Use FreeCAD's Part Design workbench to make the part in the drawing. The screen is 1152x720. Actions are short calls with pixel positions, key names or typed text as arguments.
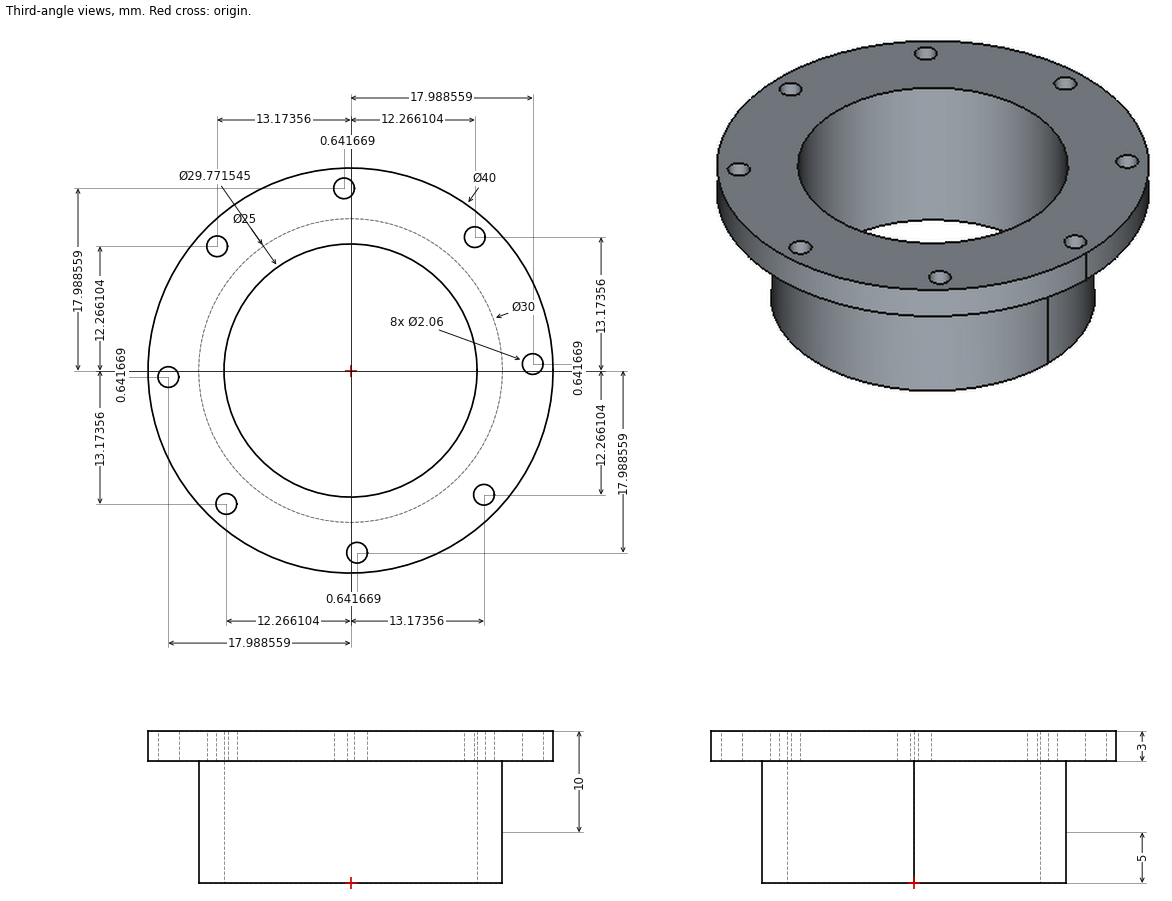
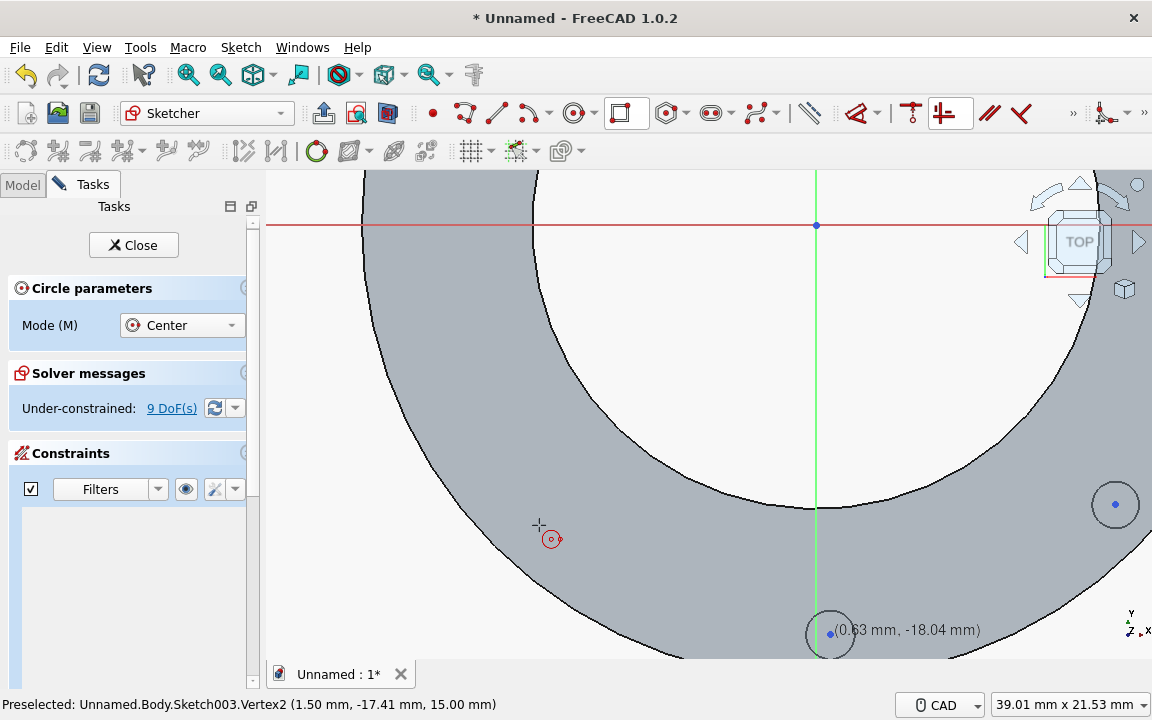
click(538, 524)
click(554, 508)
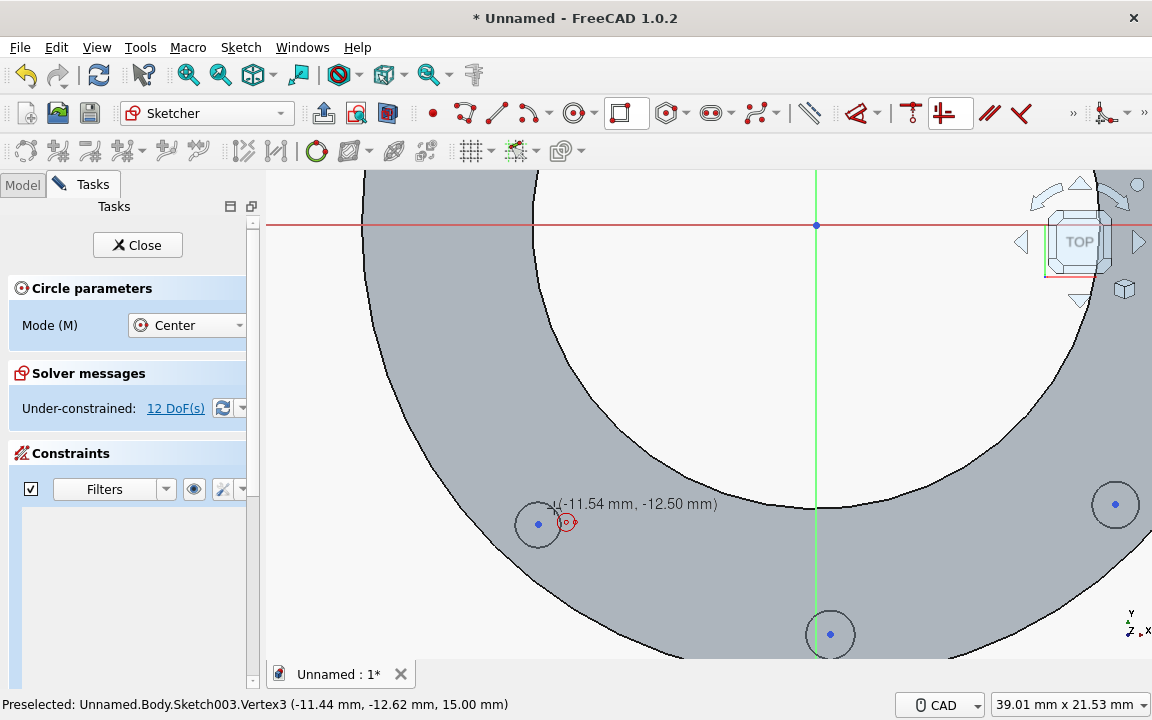
click(408, 240)
click(424, 256)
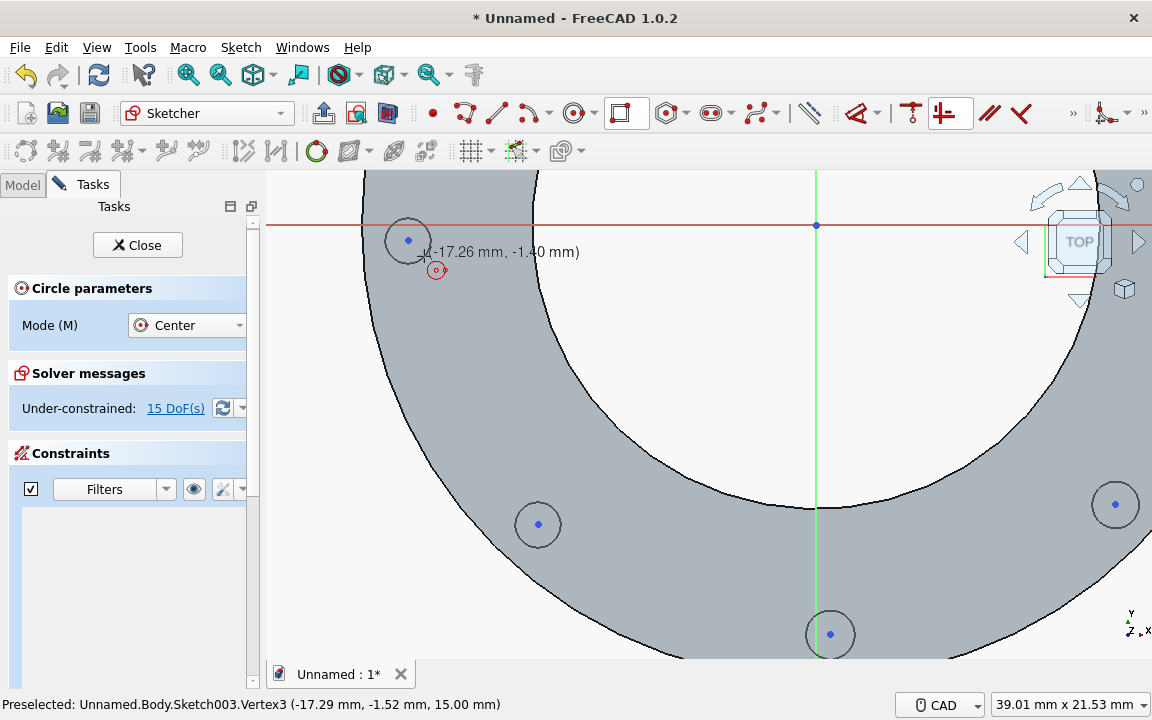
scroll(538, 525, down, 5)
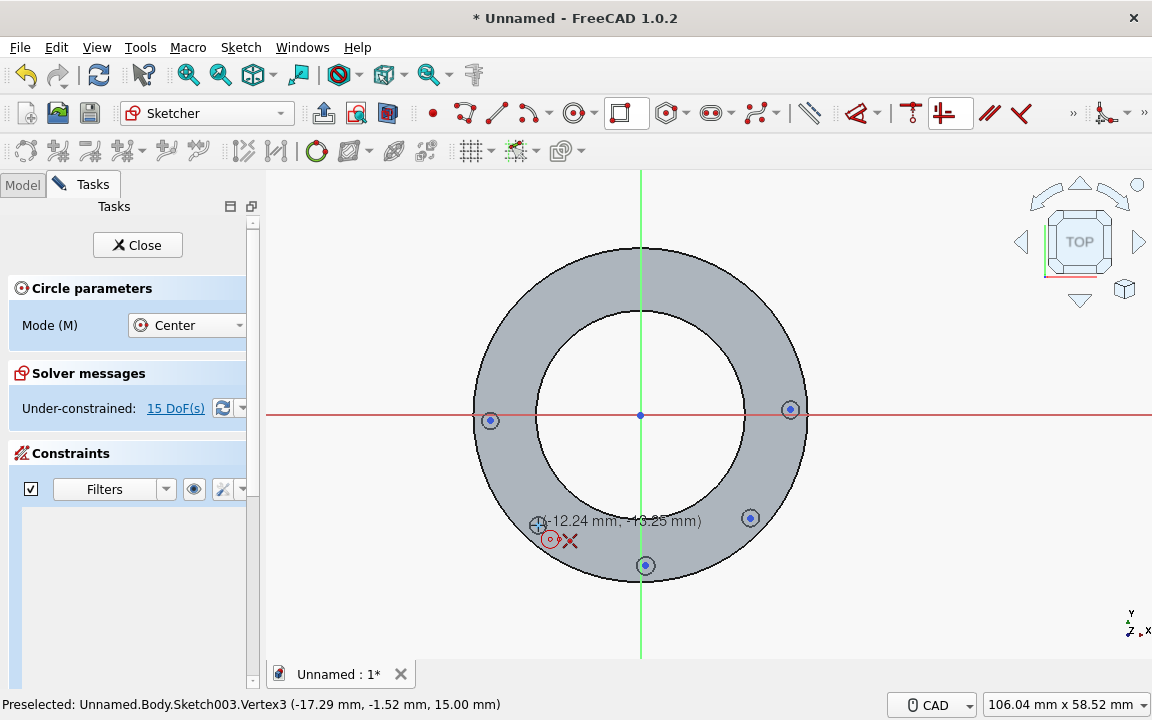
scroll(530, 313, up, 5)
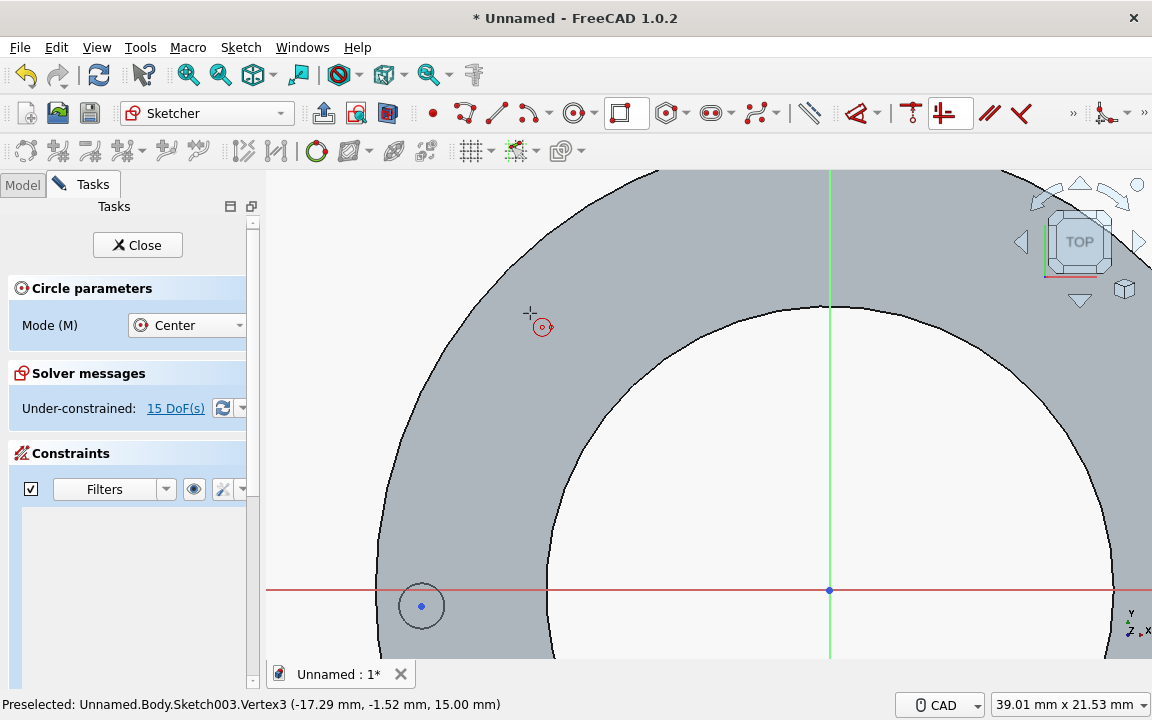
click(531, 312)
click(547, 295)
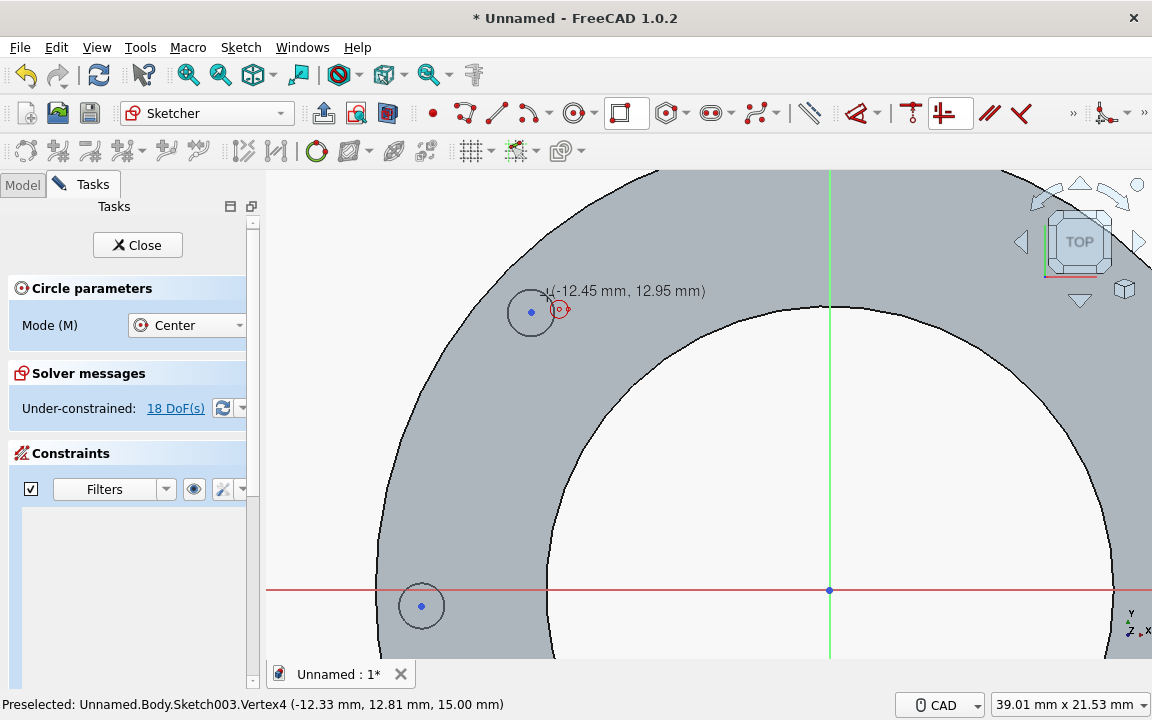
scroll(530, 312, down, 5)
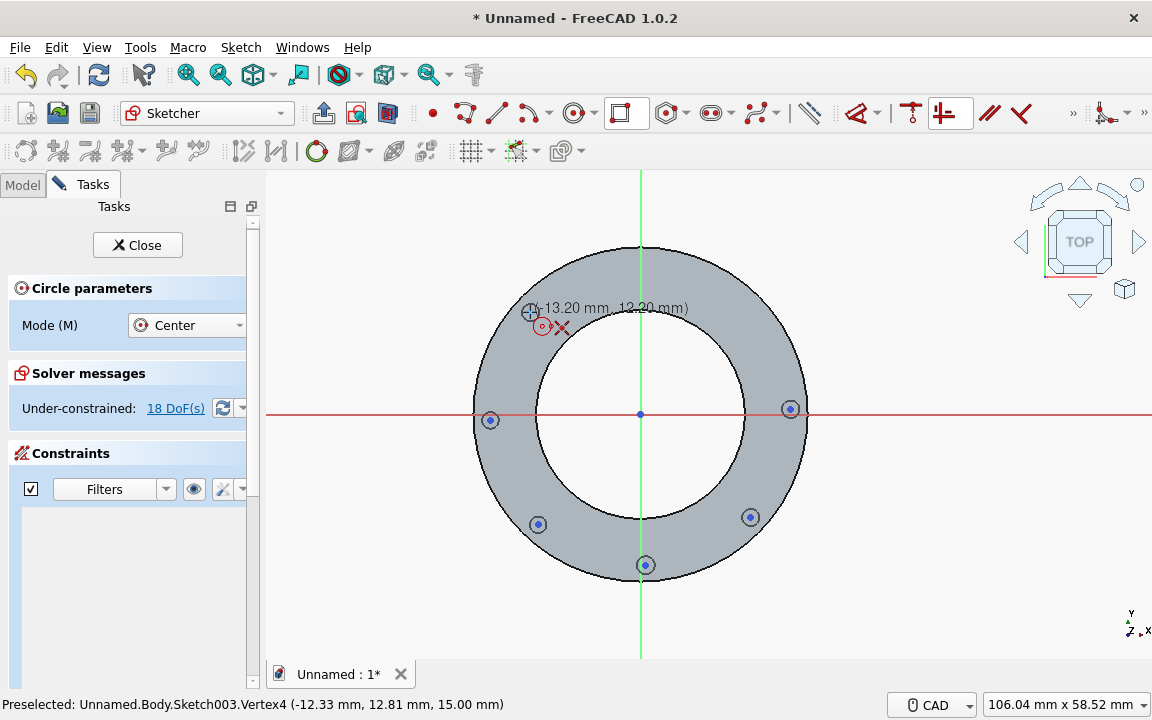
scroll(635, 264, up, 6)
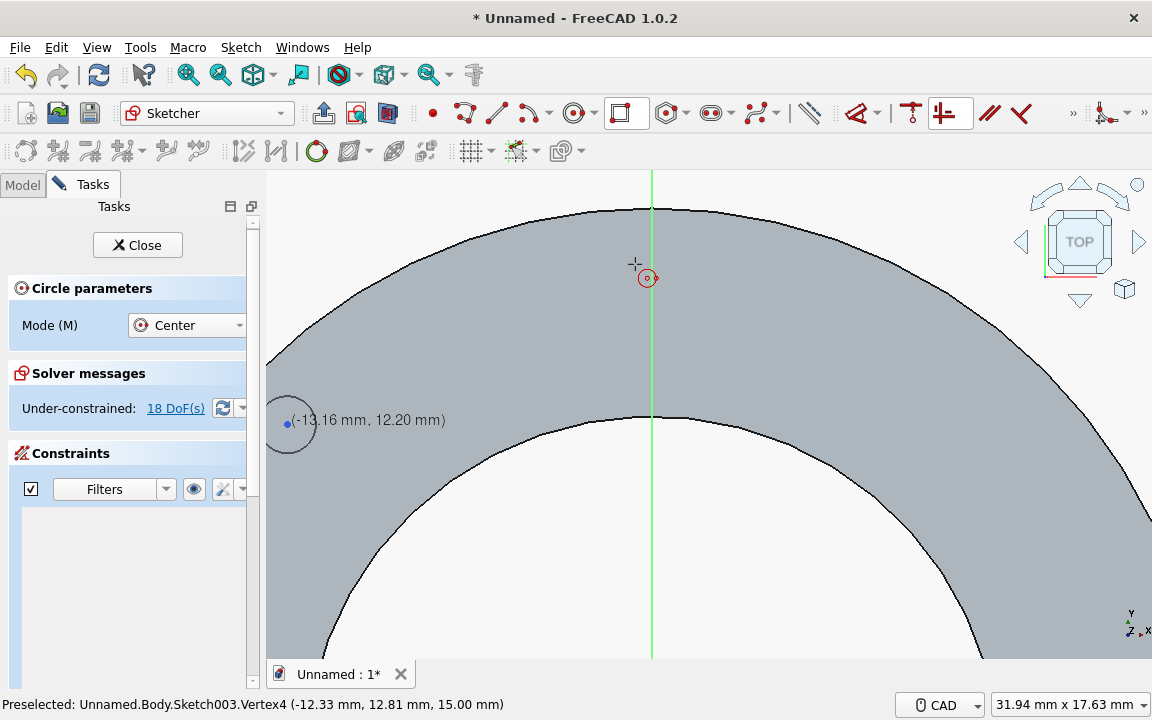
click(635, 264)
click(614, 244)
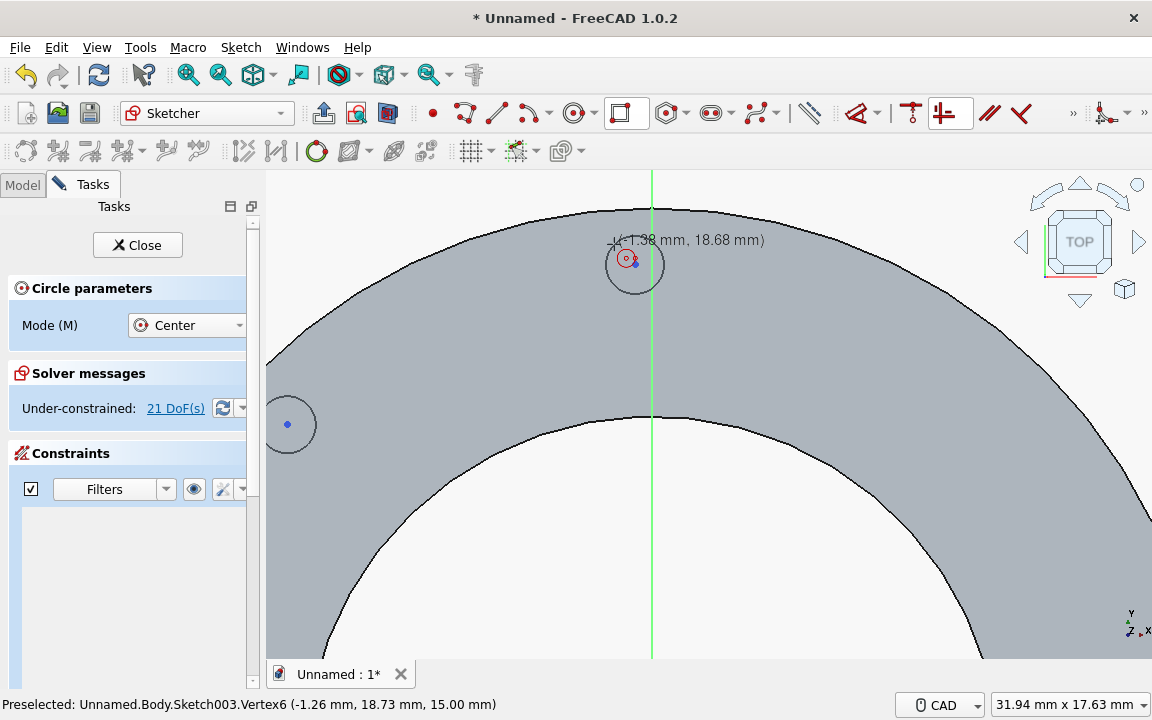
scroll(635, 264, down, 6)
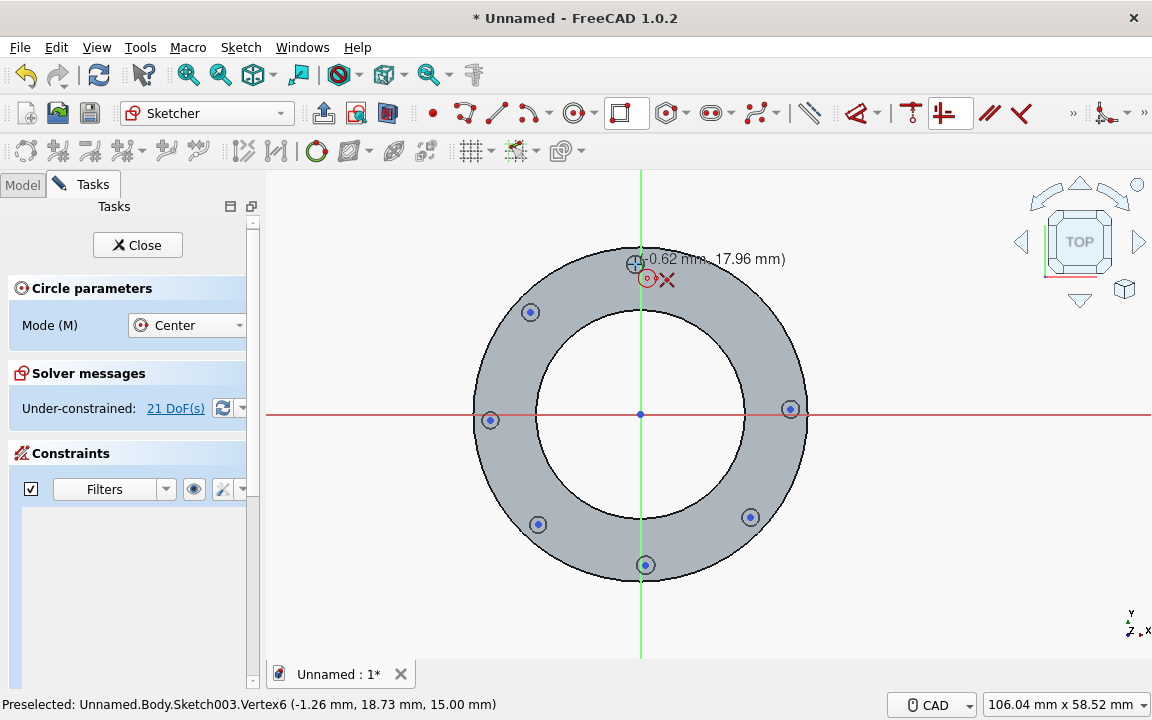
scroll(743, 304, up, 5)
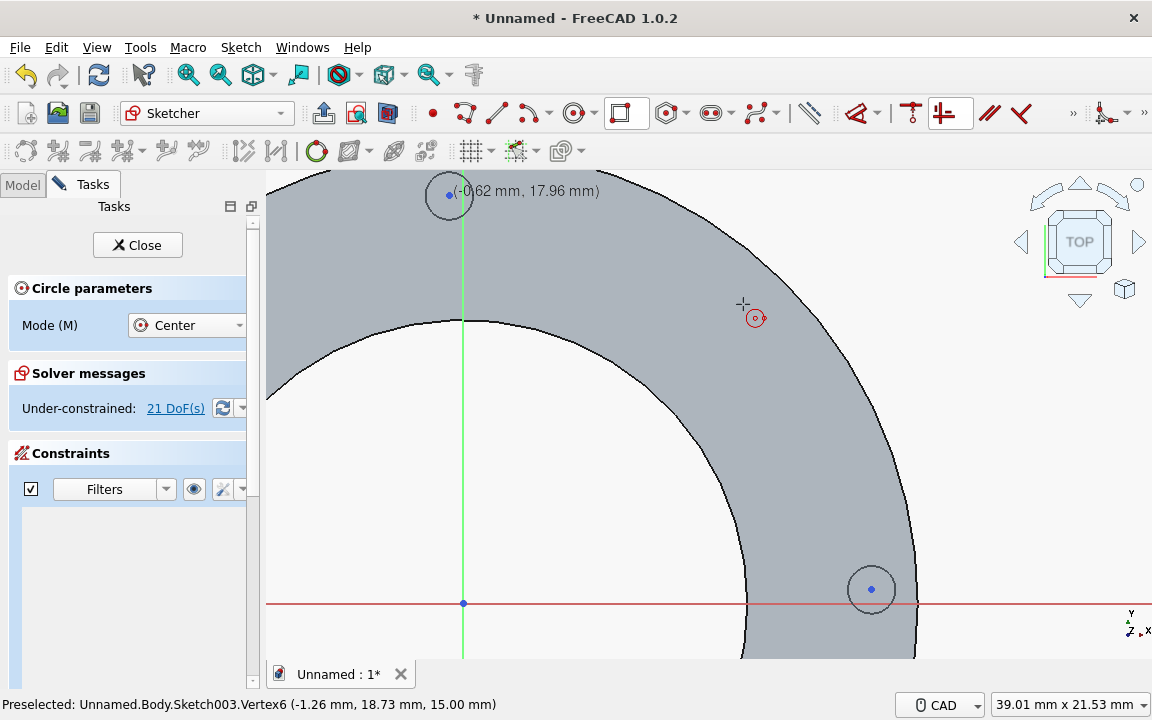
click(742, 305)
click(759, 288)
key(Escape)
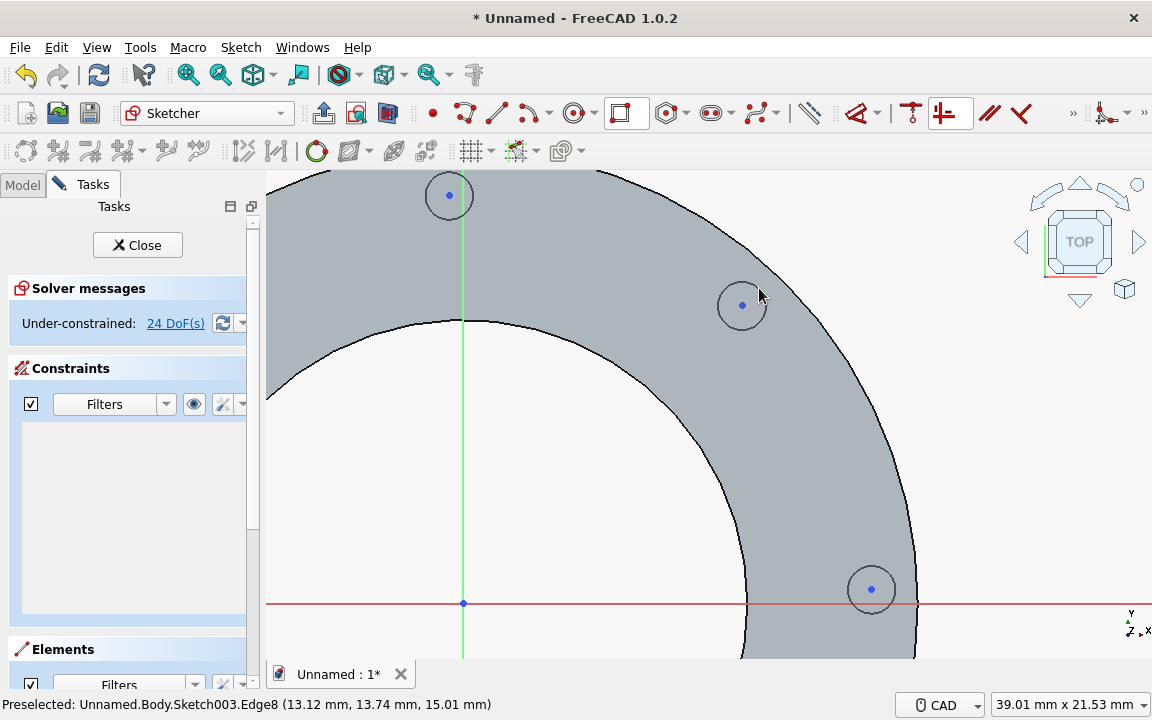
click(888, 573)